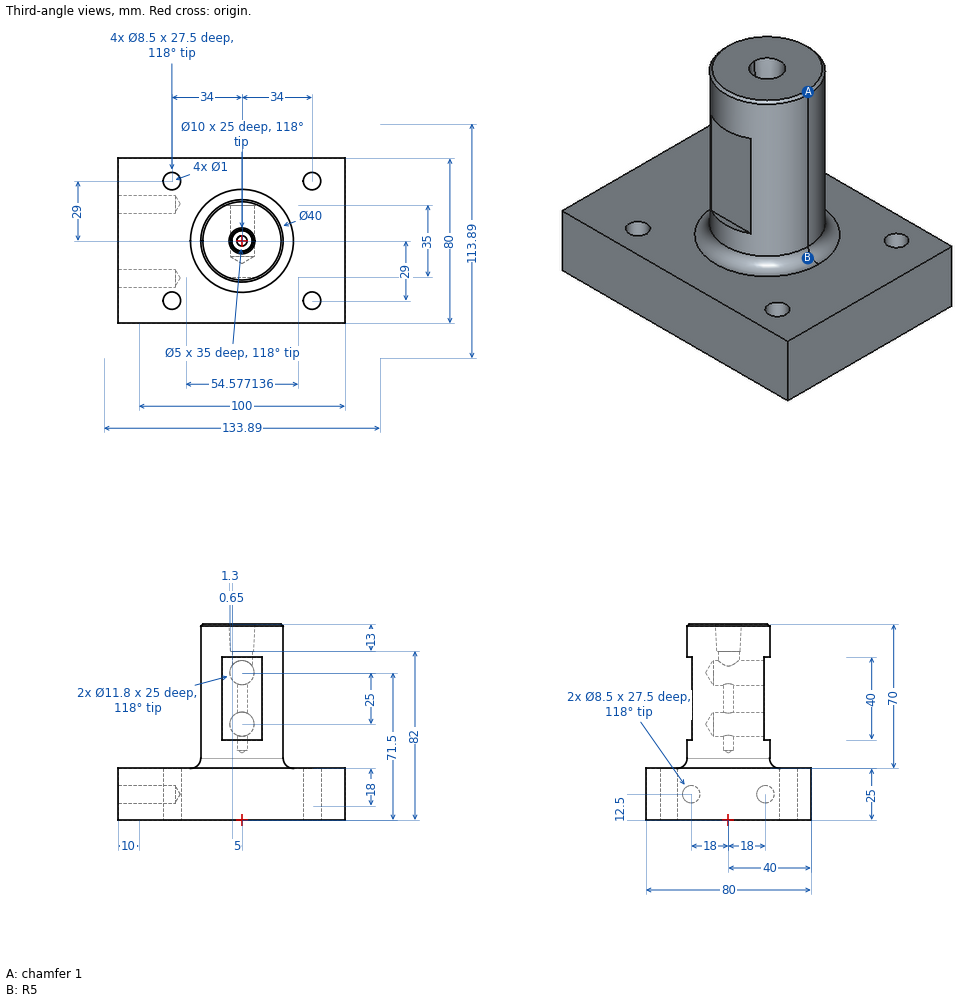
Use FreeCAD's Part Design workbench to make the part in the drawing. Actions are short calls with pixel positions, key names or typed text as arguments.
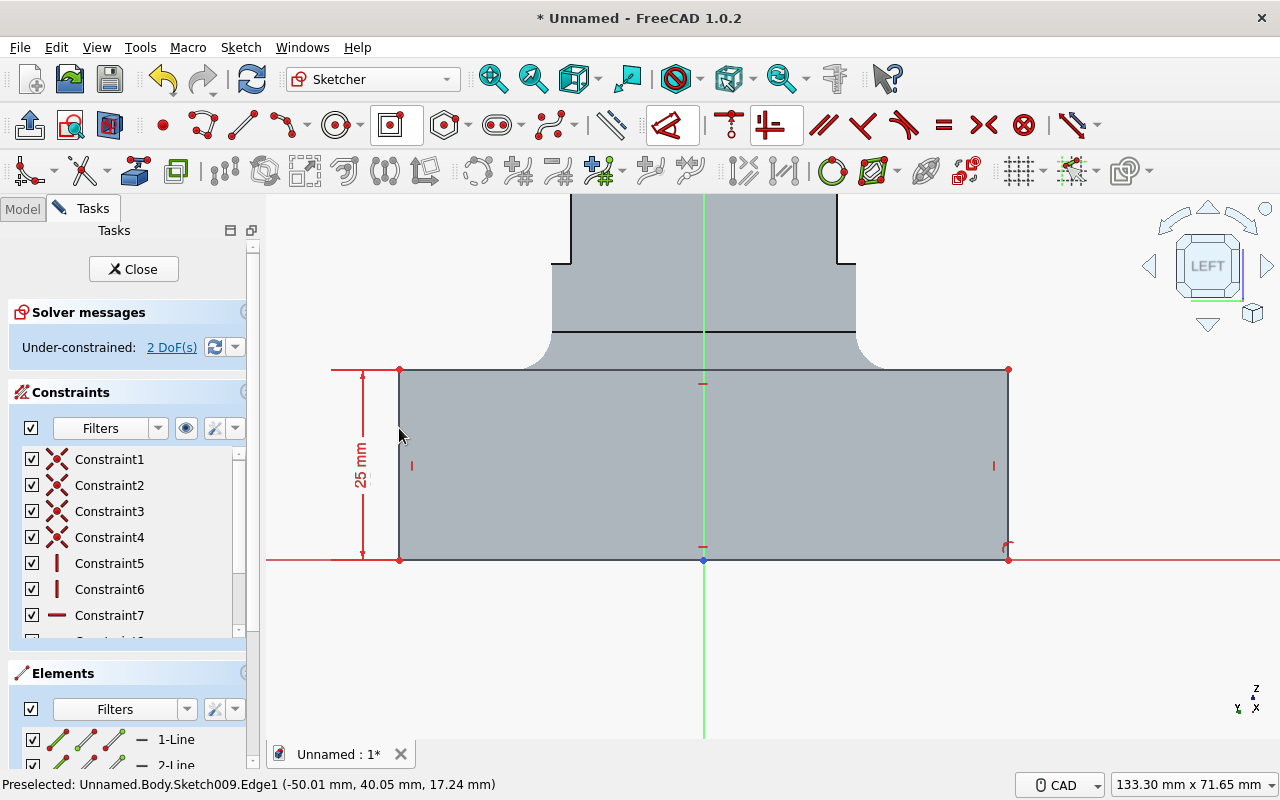
click(582, 560)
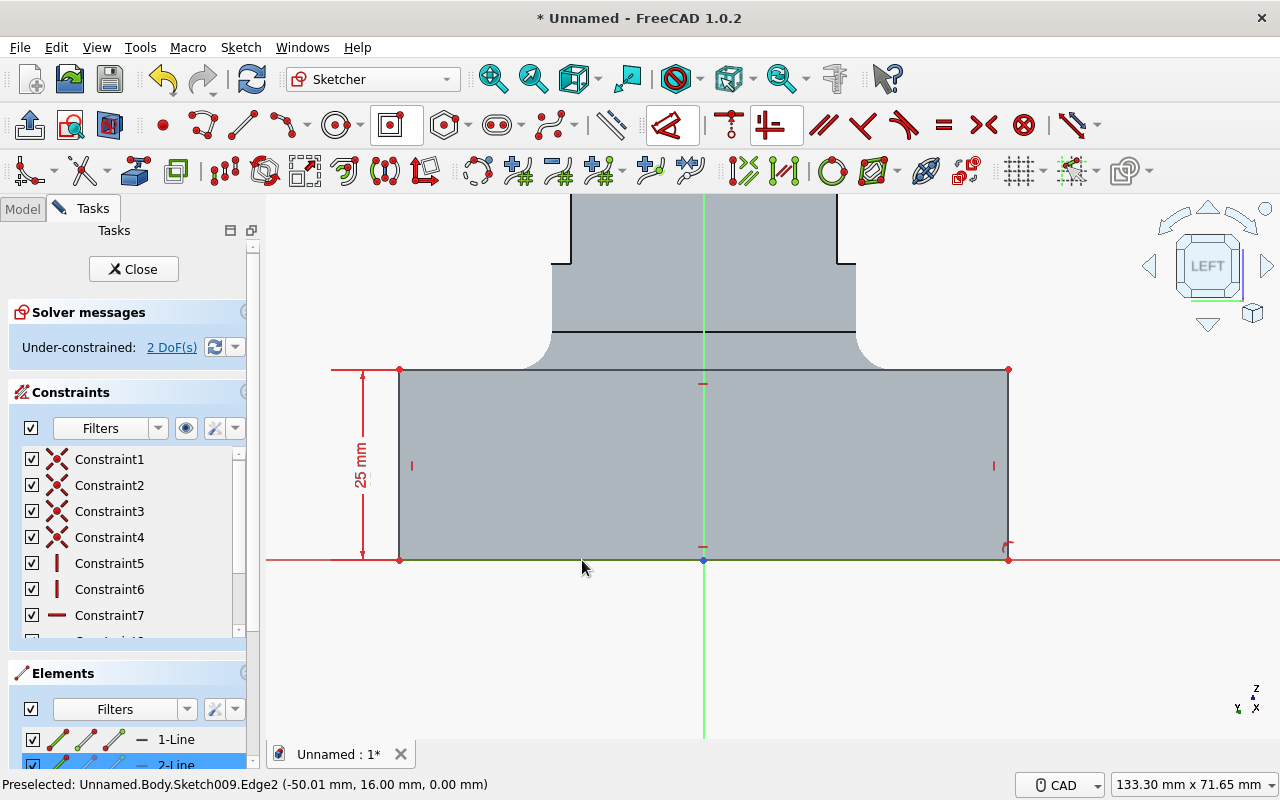
click(694, 126)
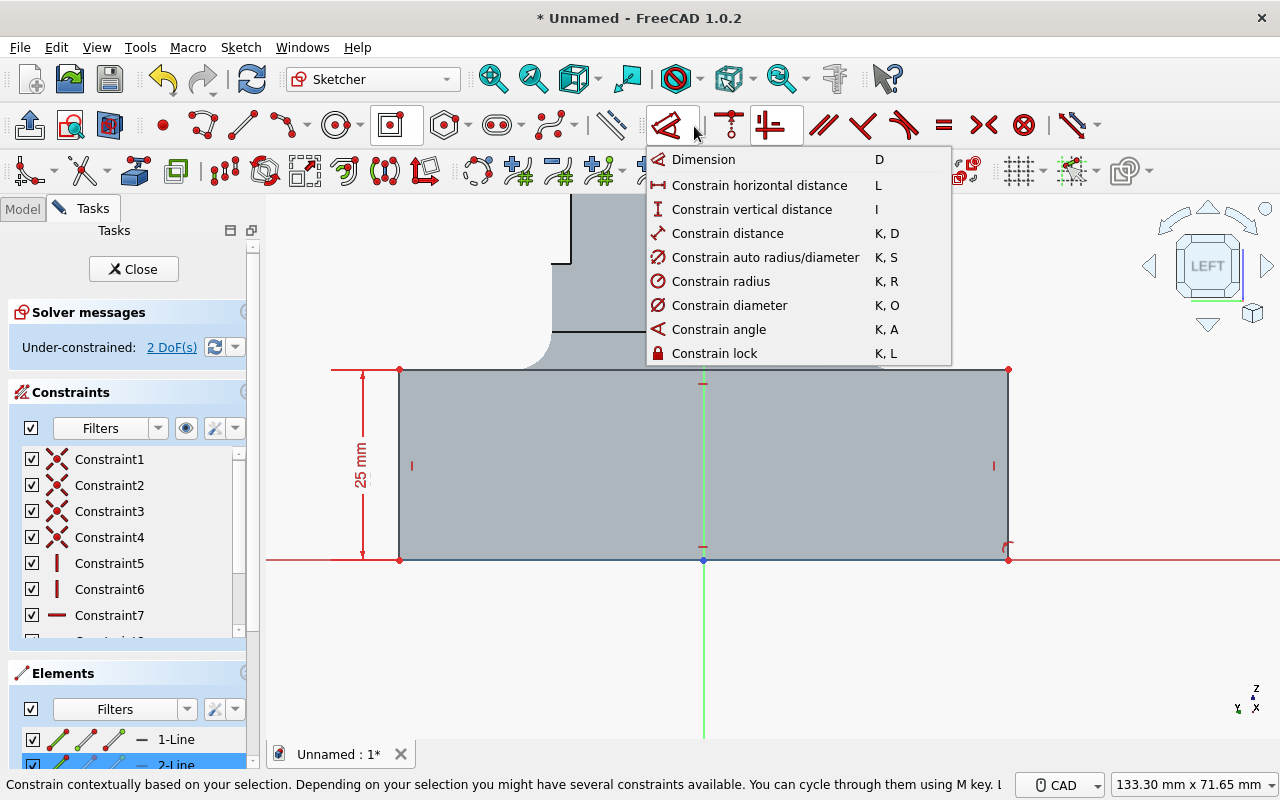
click(799, 185)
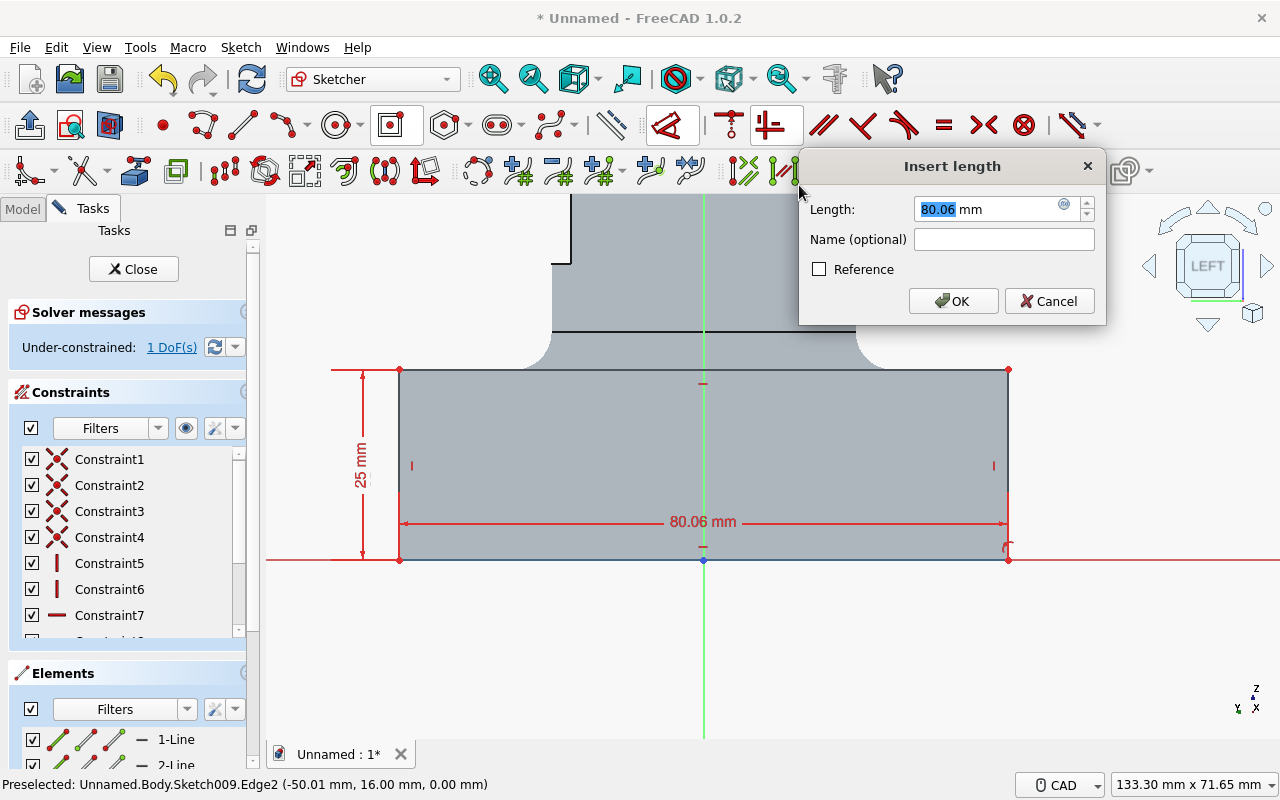
text(80)
key(Return)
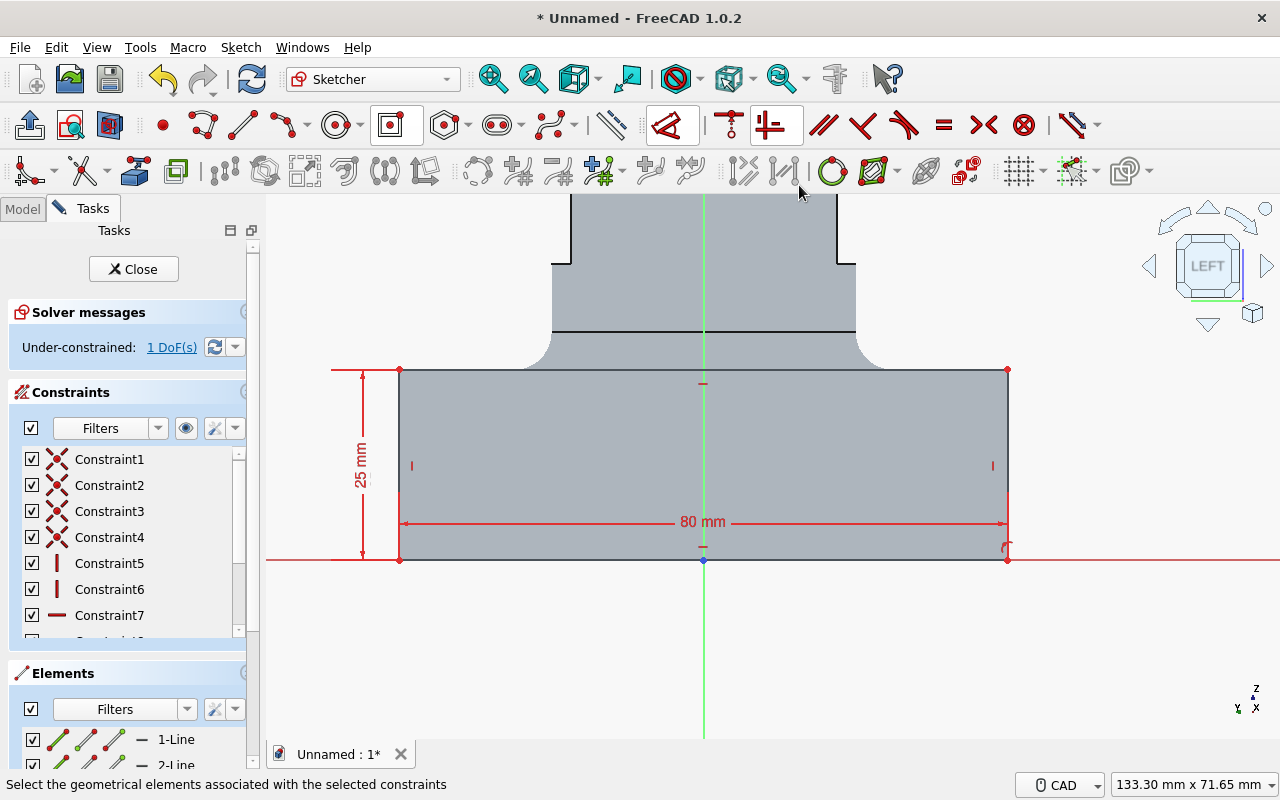
click(399, 370)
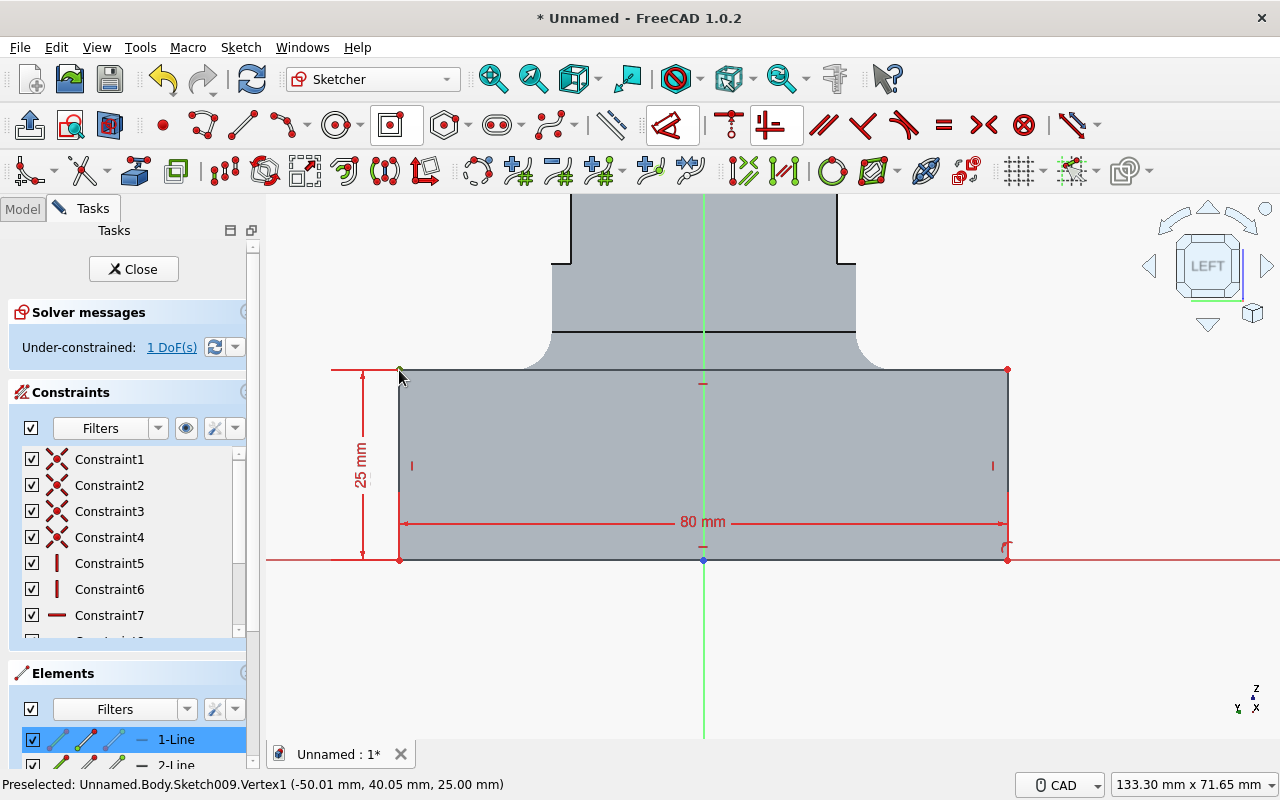
click(694, 126)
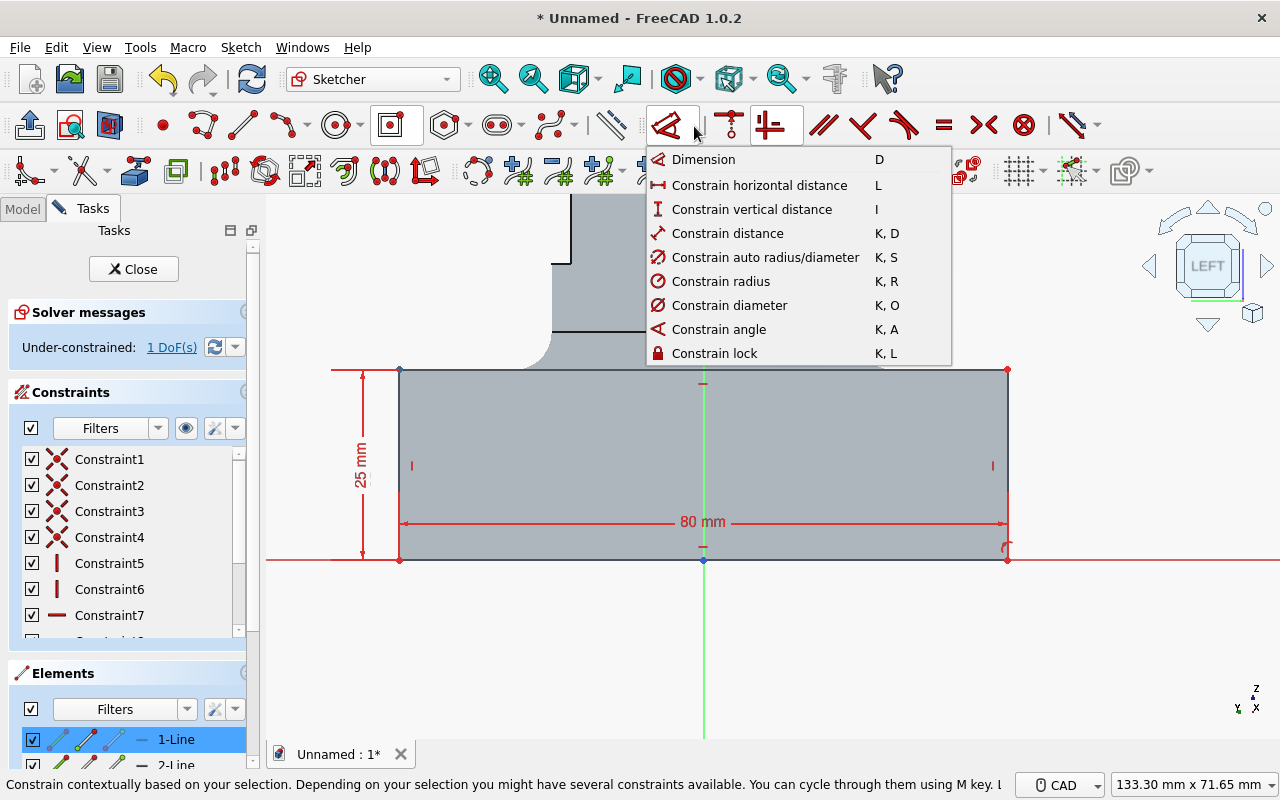
click(799, 185)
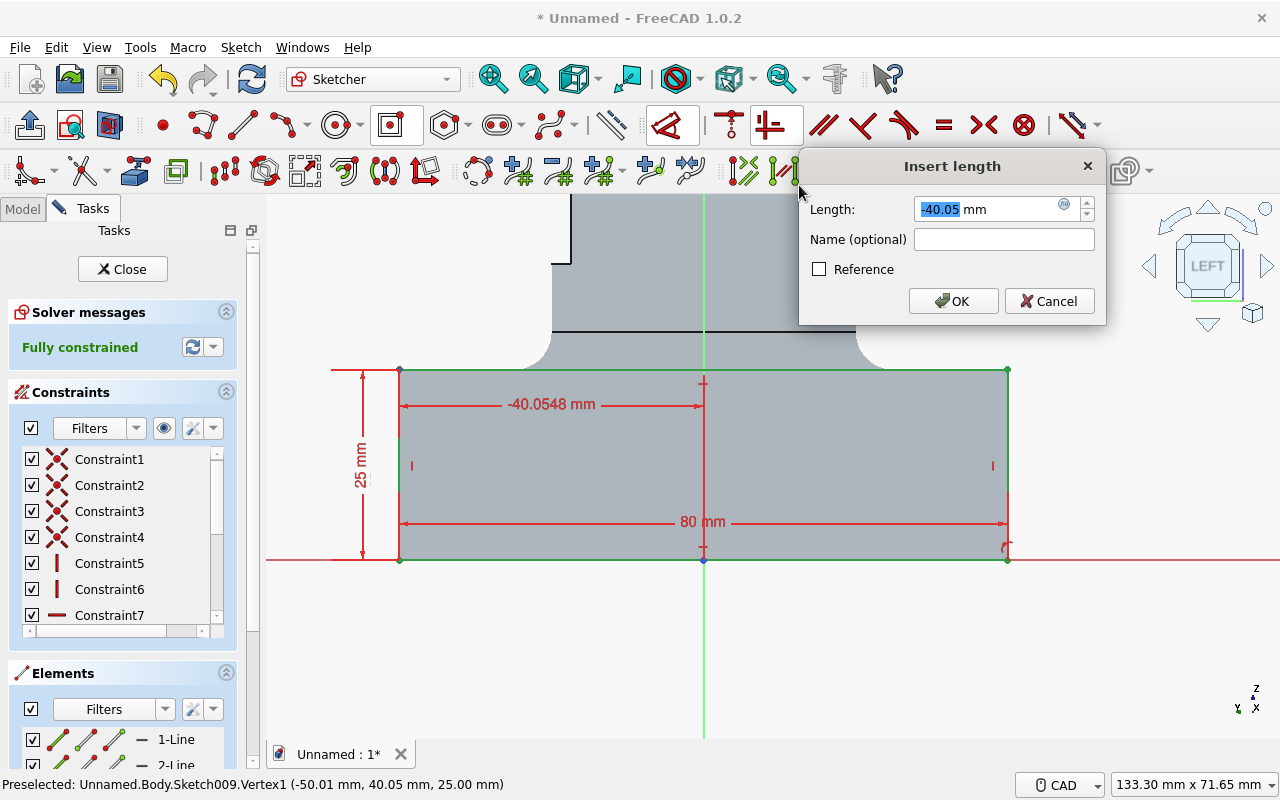
text(-40)
key(Return)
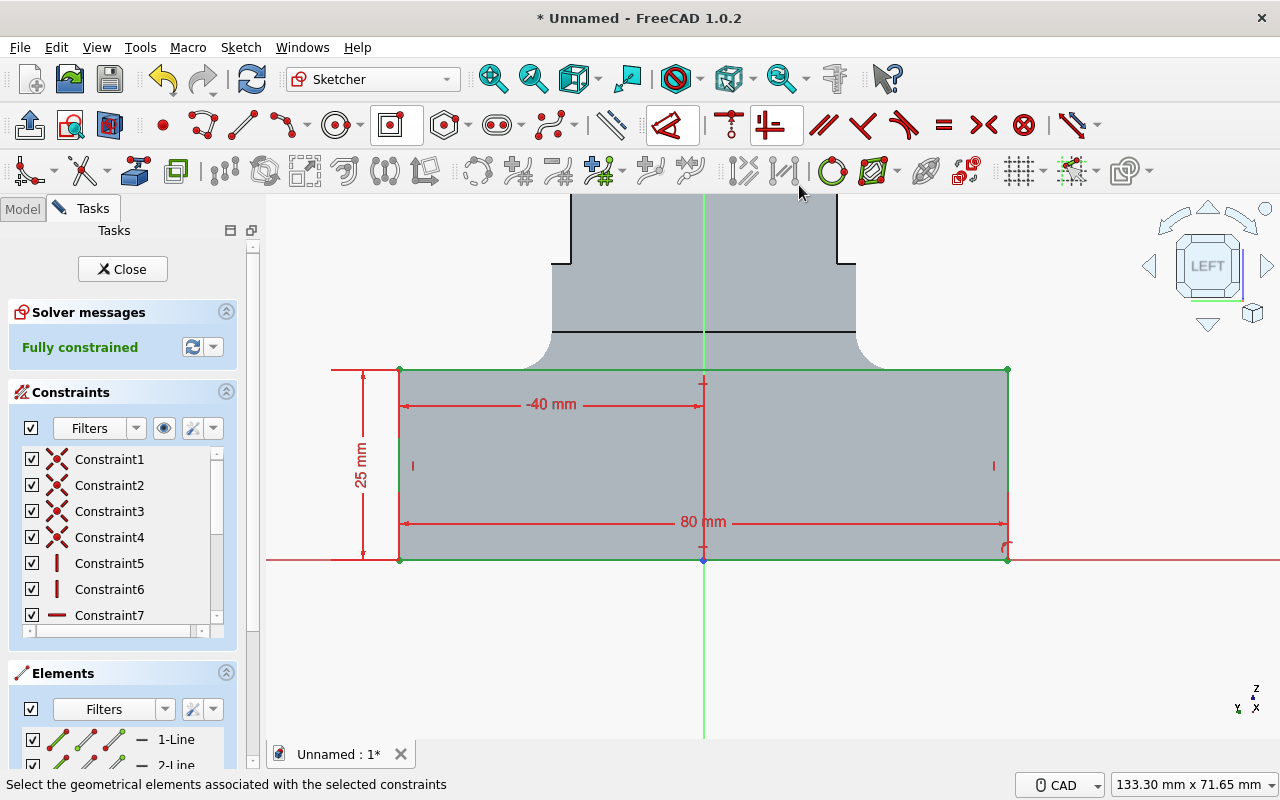
click(123, 269)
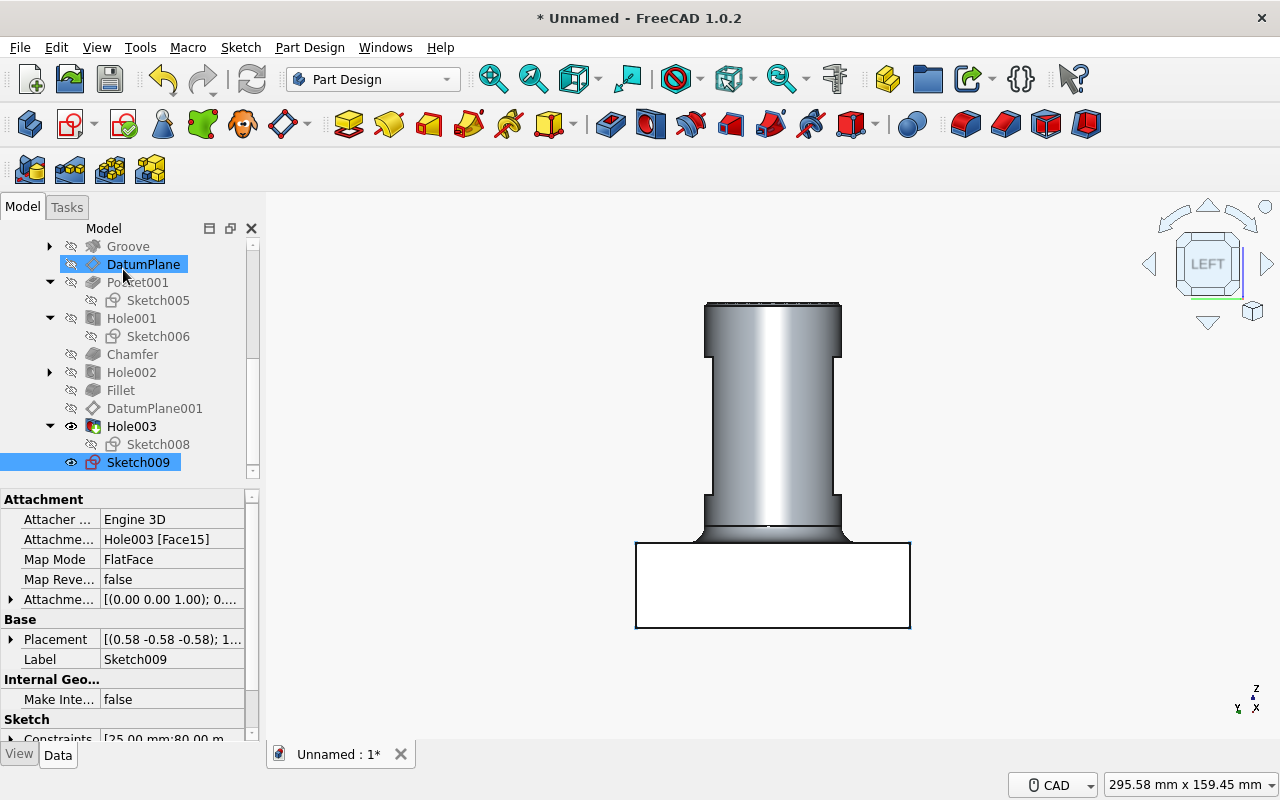
click(350, 124)